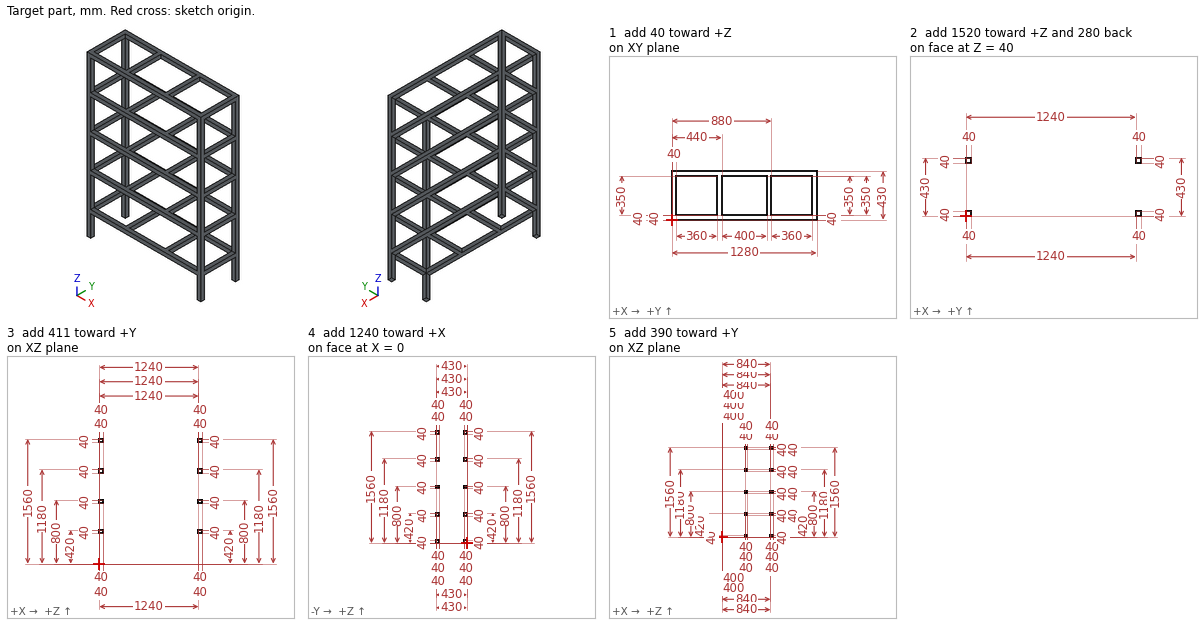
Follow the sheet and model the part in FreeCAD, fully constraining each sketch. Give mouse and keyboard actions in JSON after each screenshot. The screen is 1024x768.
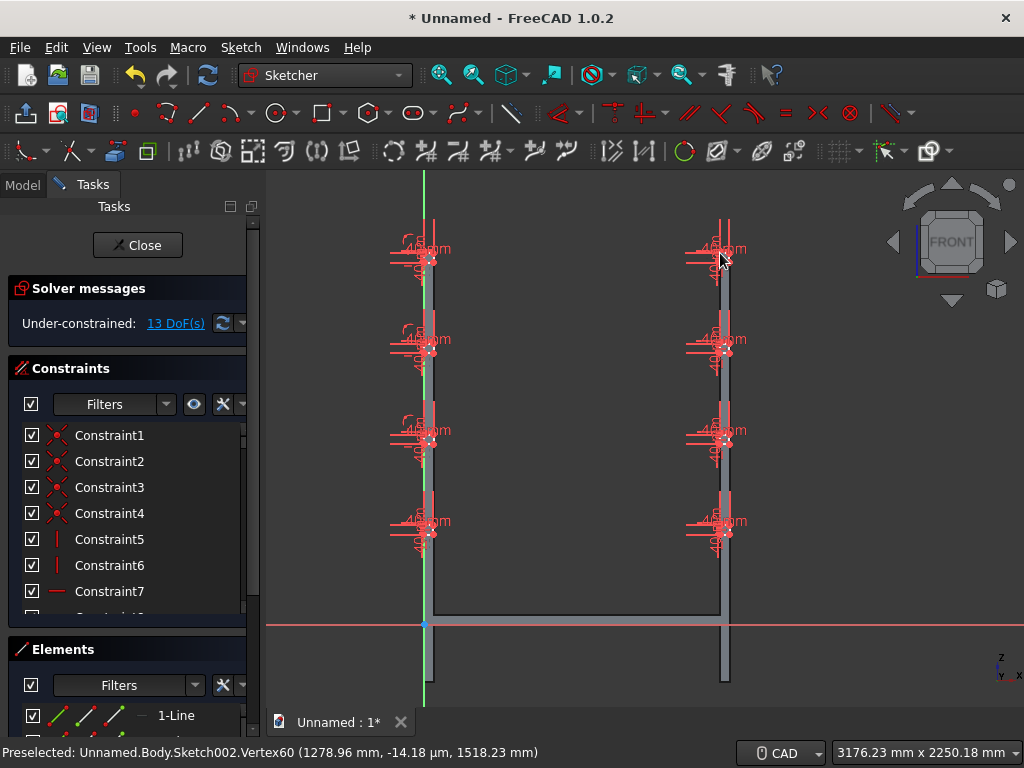
{"action": "scroll", "coordinate": [424, 525], "scroll_direction": "up", "scroll_amount": 2}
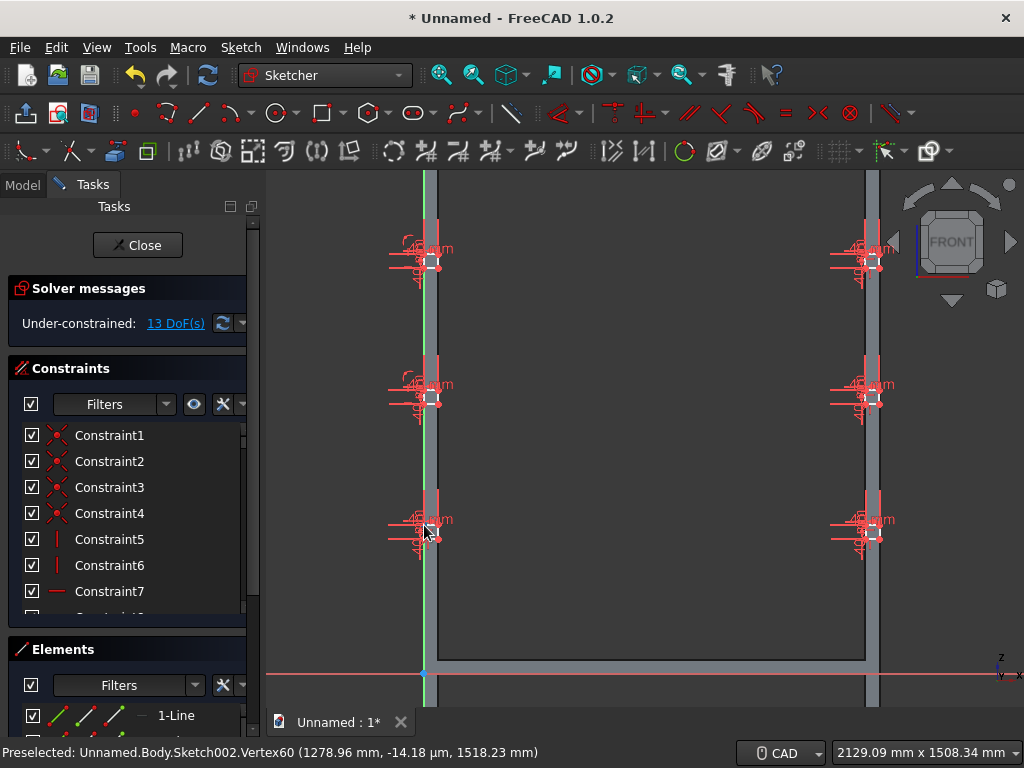
{"action": "left_click", "coordinate": [424, 525]}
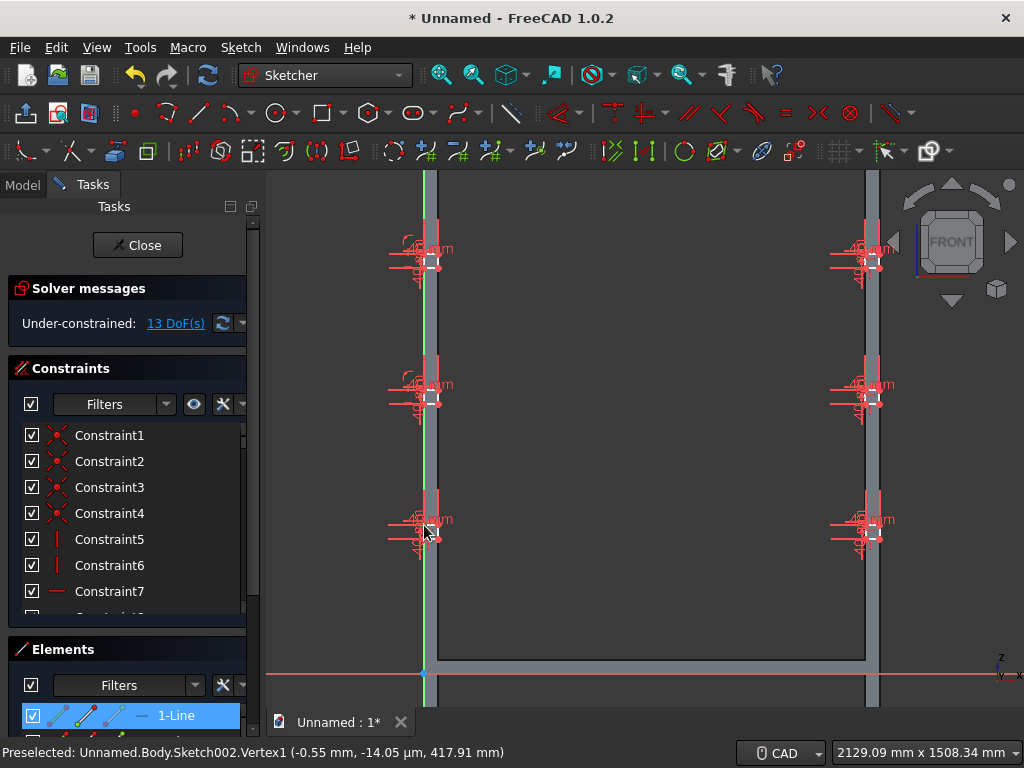
{"action": "left_click", "coordinate": [424, 610]}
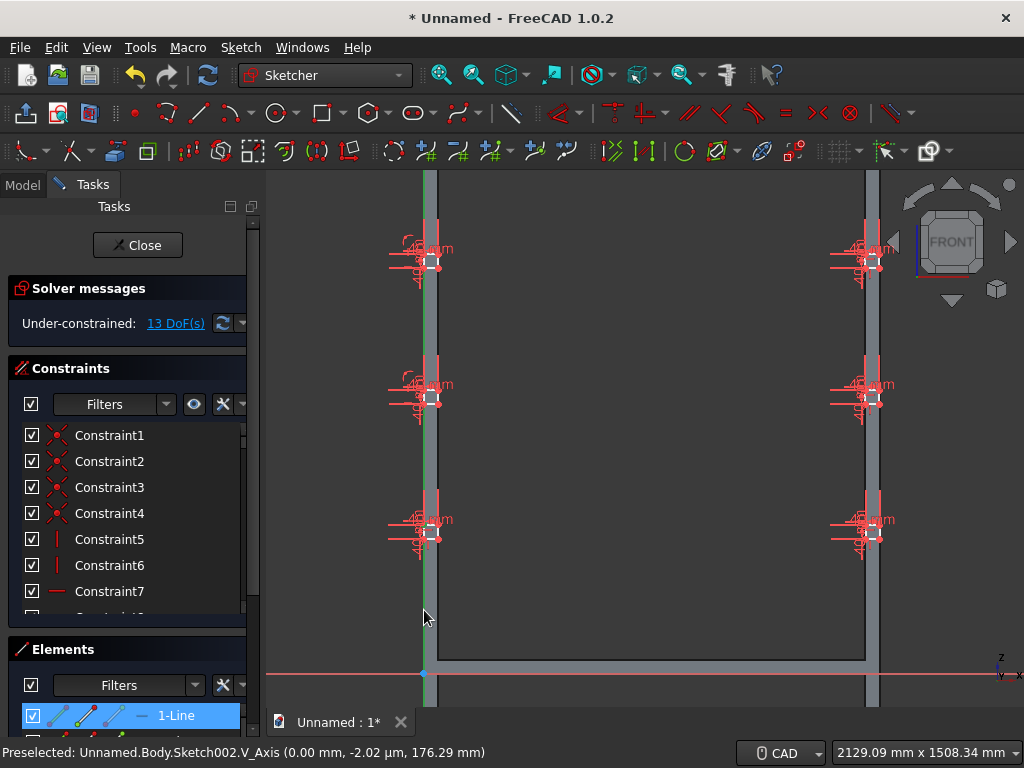
{"action": "left_click", "coordinate": [614, 114]}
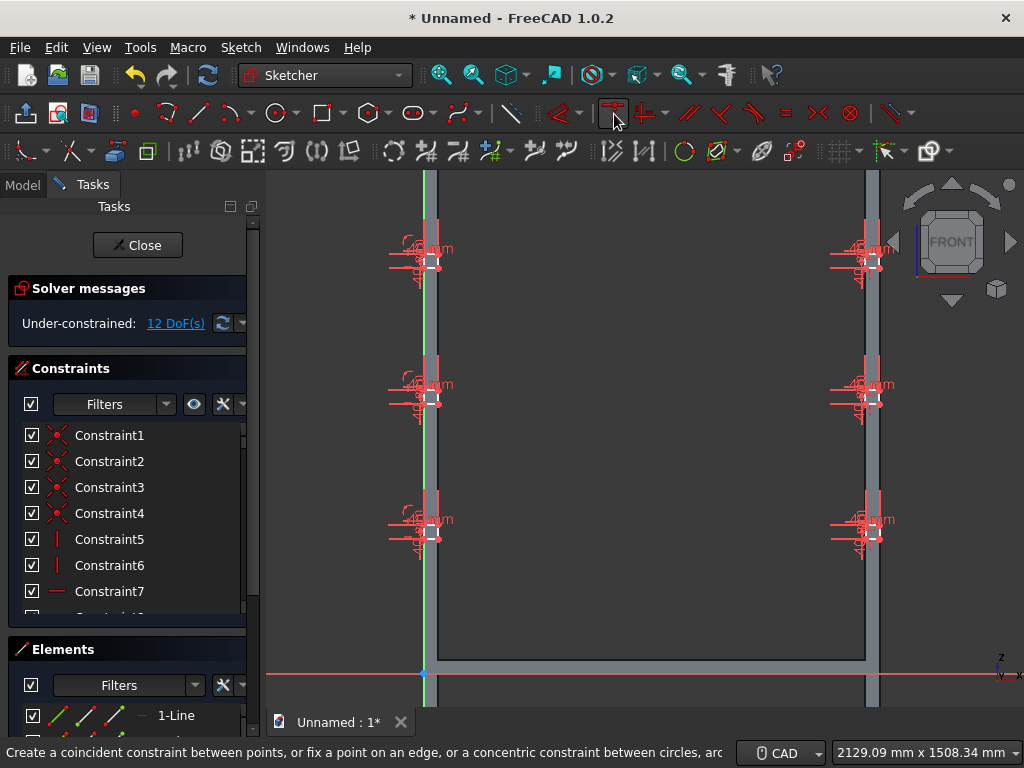
{"action": "left_click", "coordinate": [558, 114]}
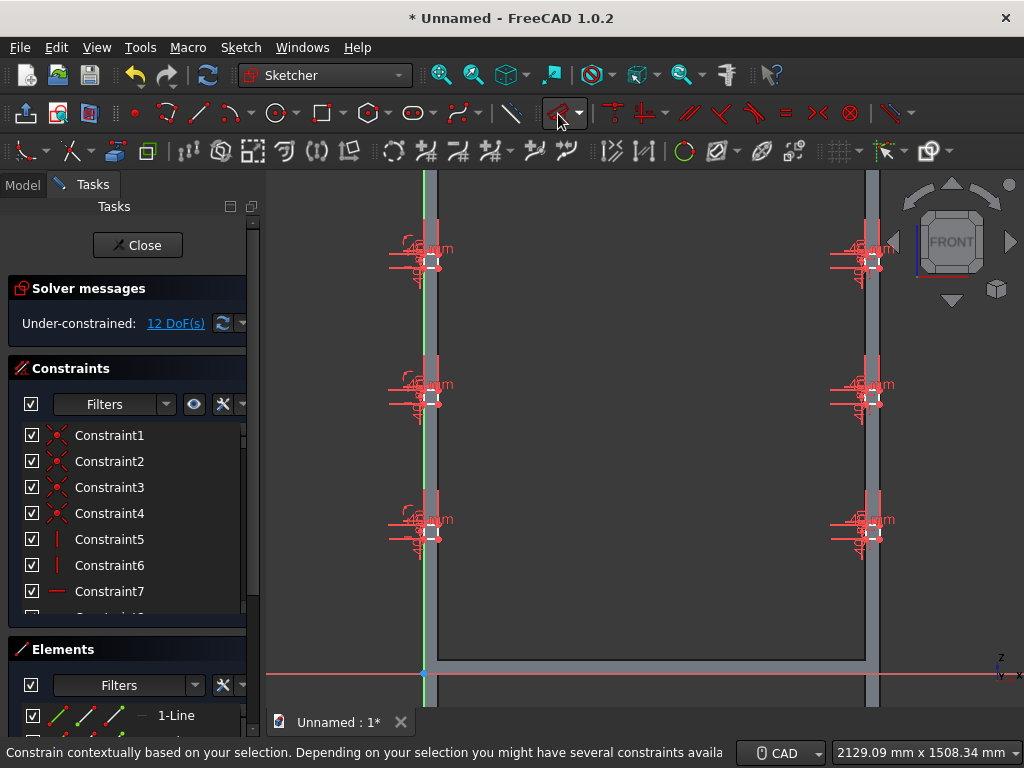
{"action": "left_click", "coordinate": [424, 525]}
{"action": "left_click", "coordinate": [390, 599]}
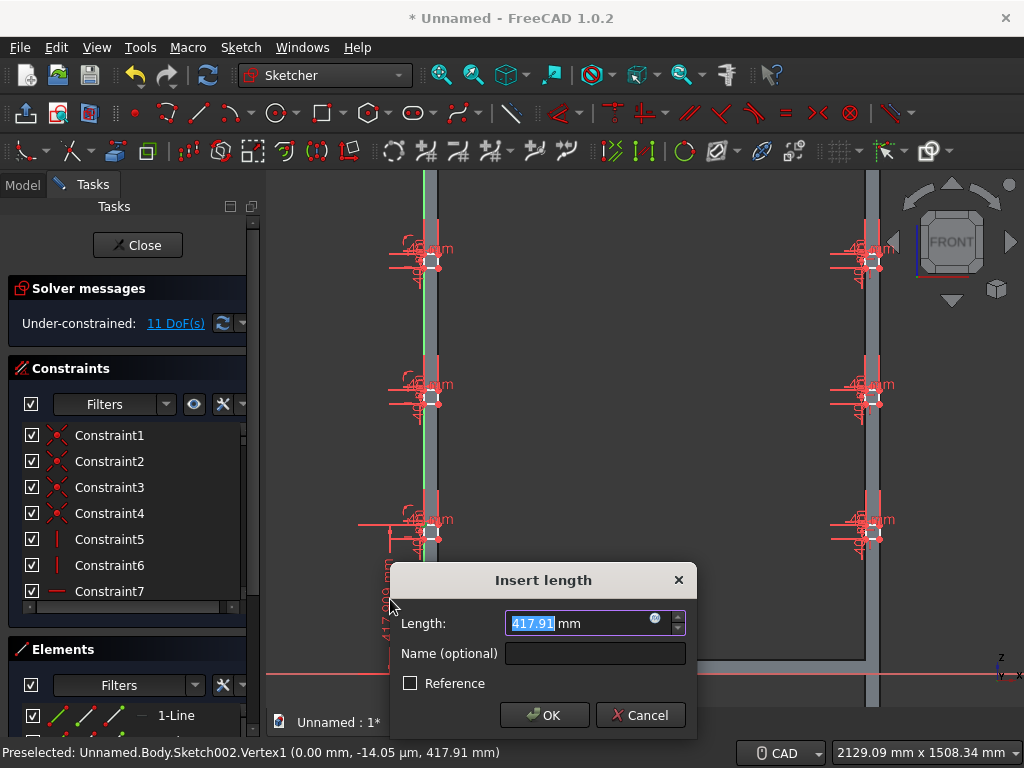
{"action": "type", "text": "420"}
{"action": "key", "text": "Return"}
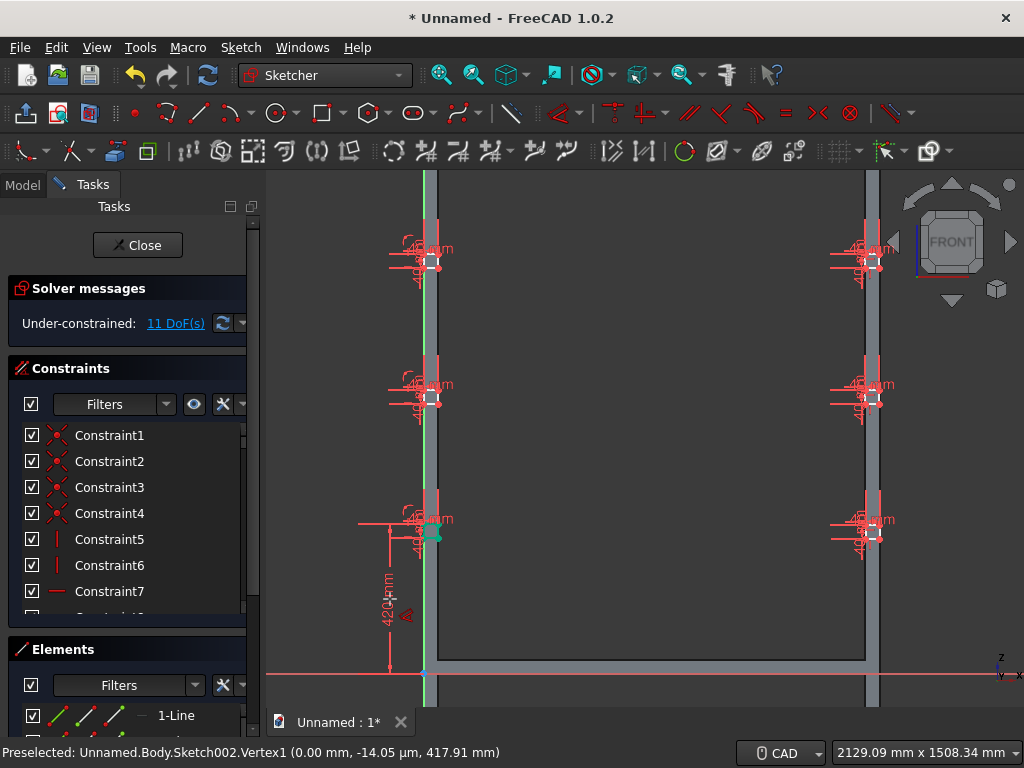
{"action": "scroll", "coordinate": [423, 525], "scroll_direction": "down", "scroll_amount": 2}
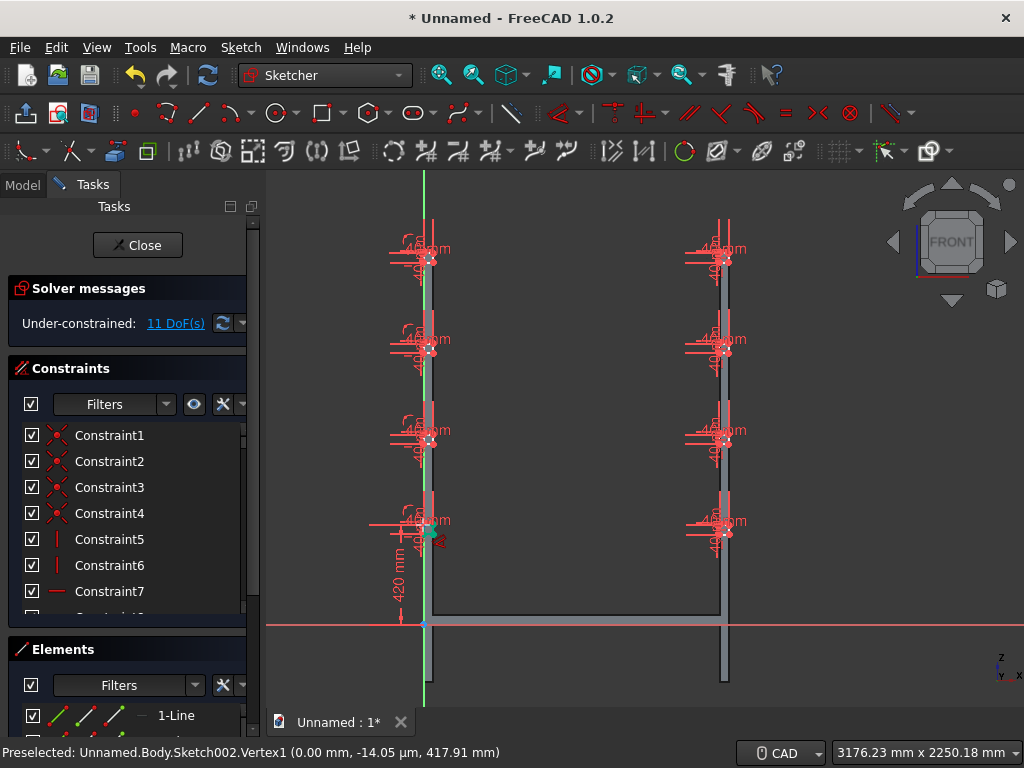
{"action": "scroll", "coordinate": [720, 525], "scroll_direction": "up", "scroll_amount": 2}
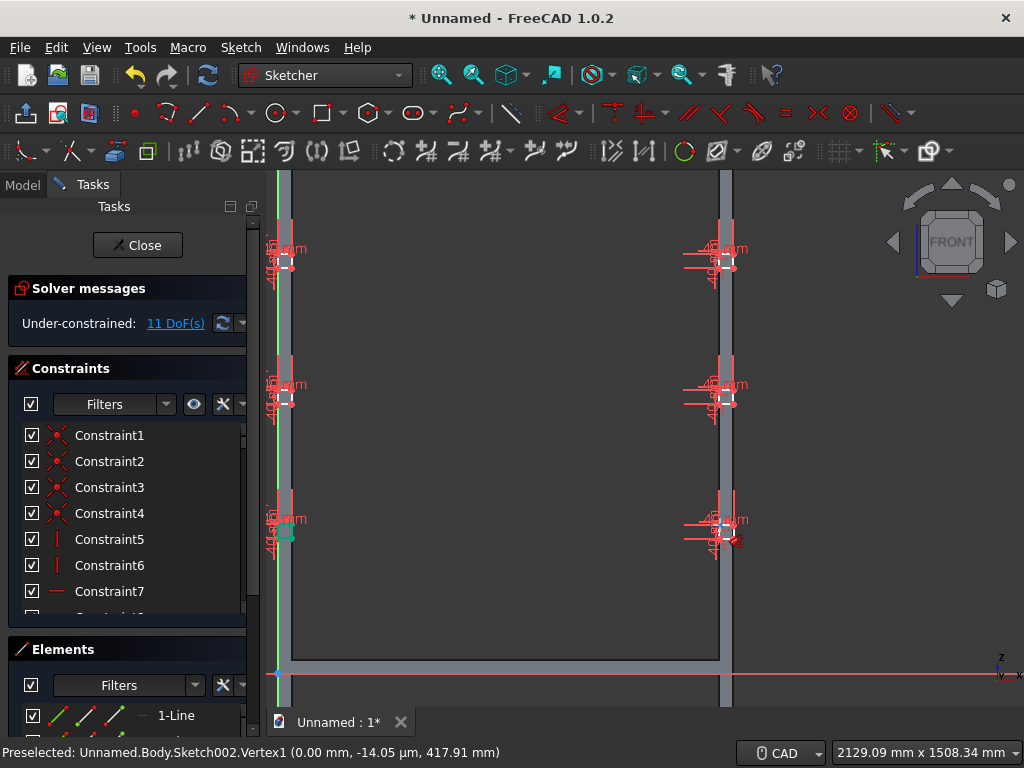
{"action": "left_click", "coordinate": [719, 525]}
{"action": "left_click", "coordinate": [753, 599]}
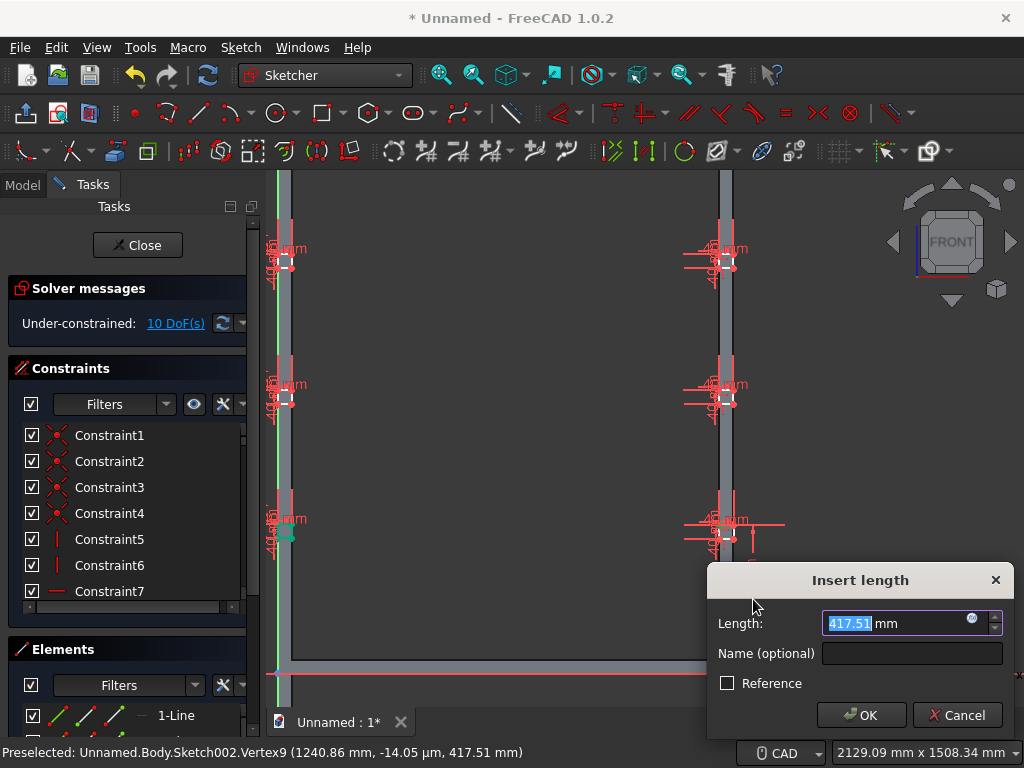
{"action": "type", "text": "420"}
{"action": "key", "text": "Return"}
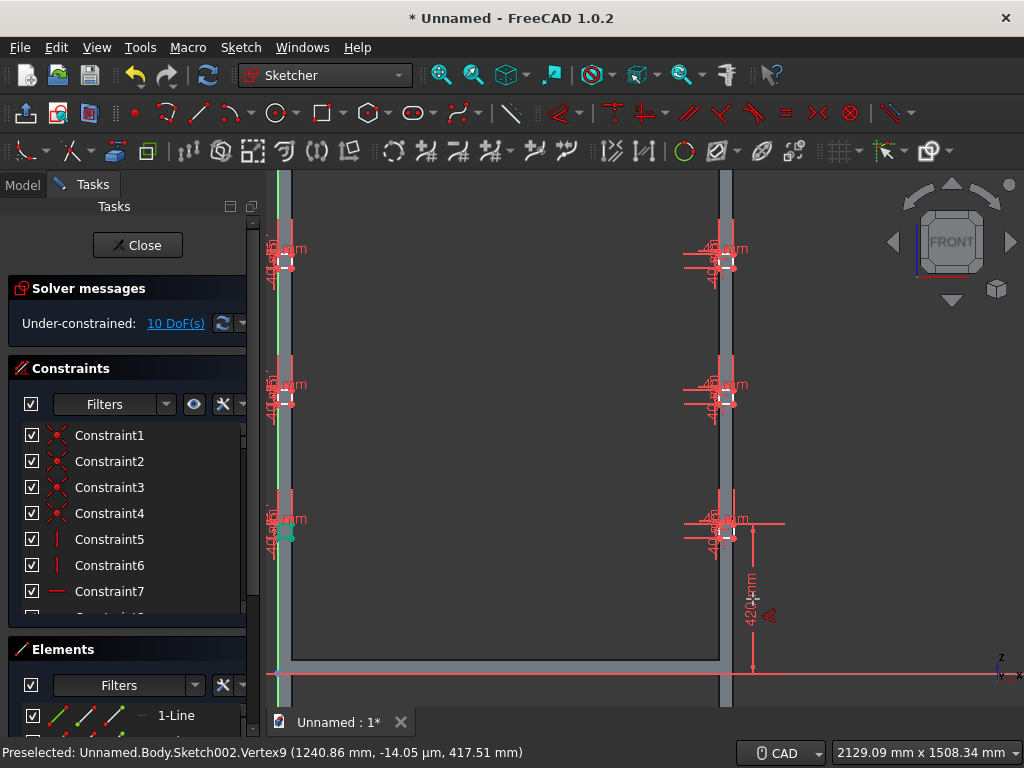
{"action": "scroll", "coordinate": [721, 525], "scroll_direction": "down", "scroll_amount": 2}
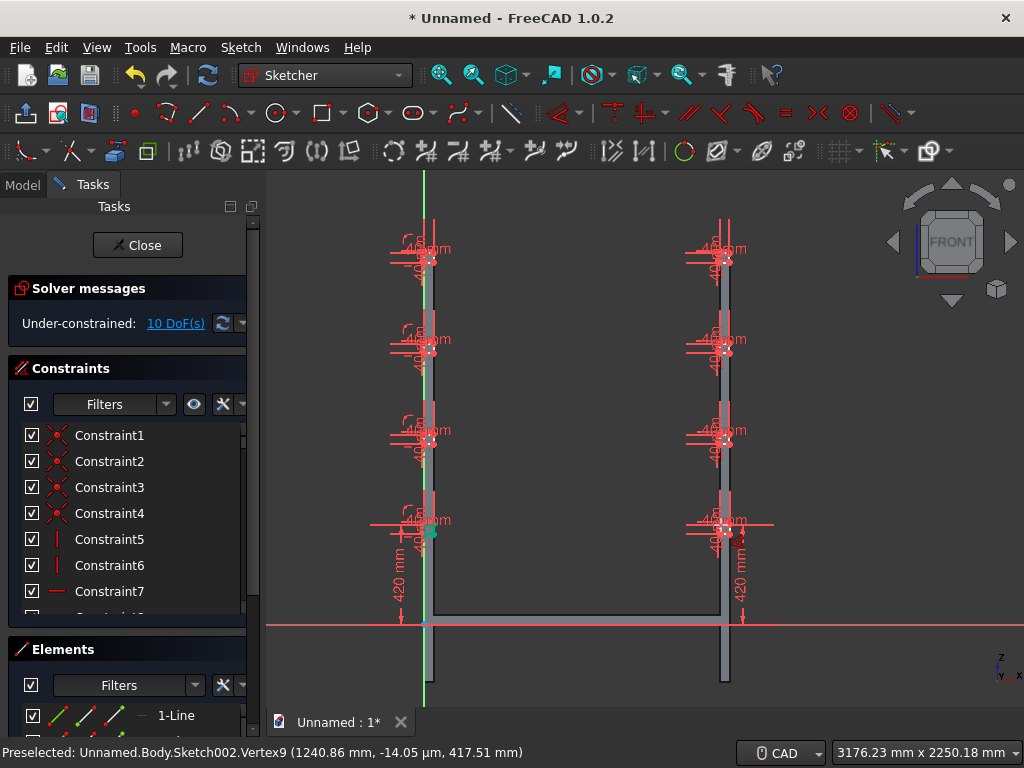
{"action": "scroll", "coordinate": [424, 435], "scroll_direction": "up", "scroll_amount": 2}